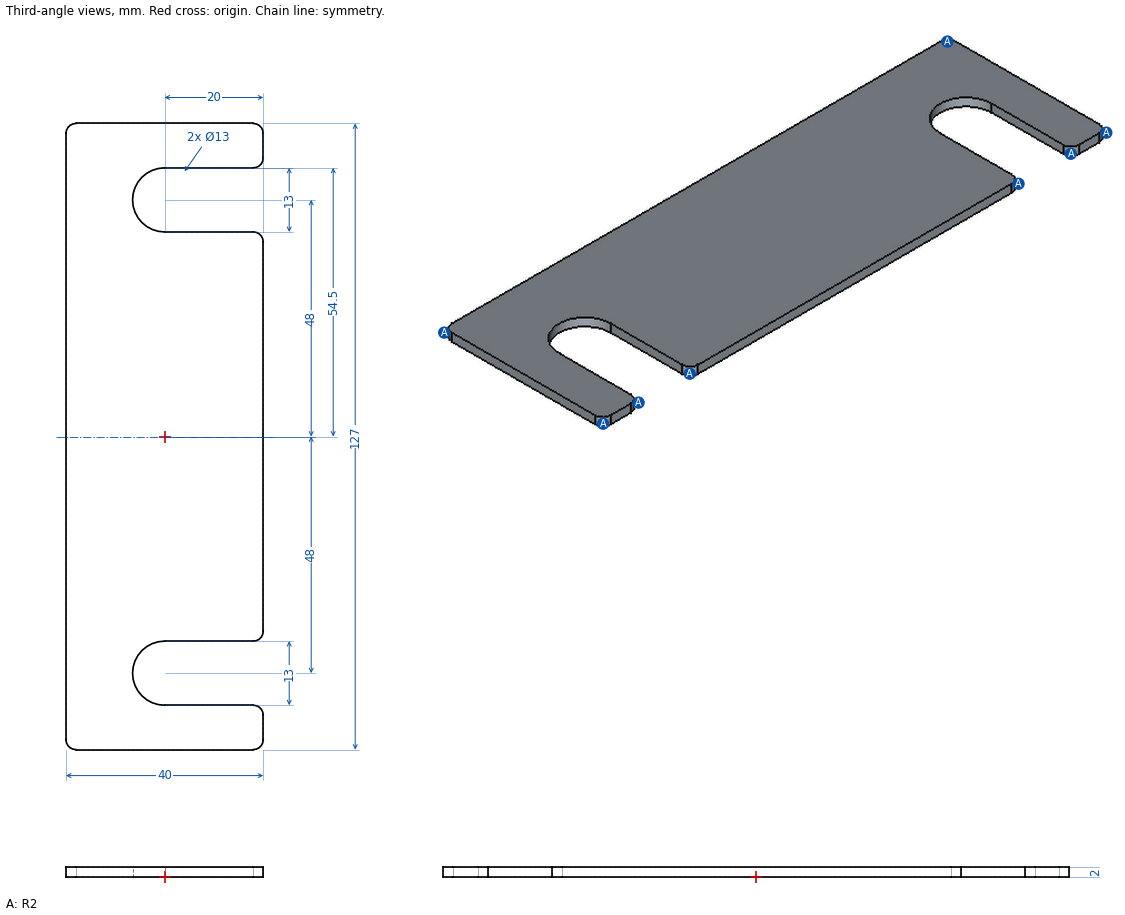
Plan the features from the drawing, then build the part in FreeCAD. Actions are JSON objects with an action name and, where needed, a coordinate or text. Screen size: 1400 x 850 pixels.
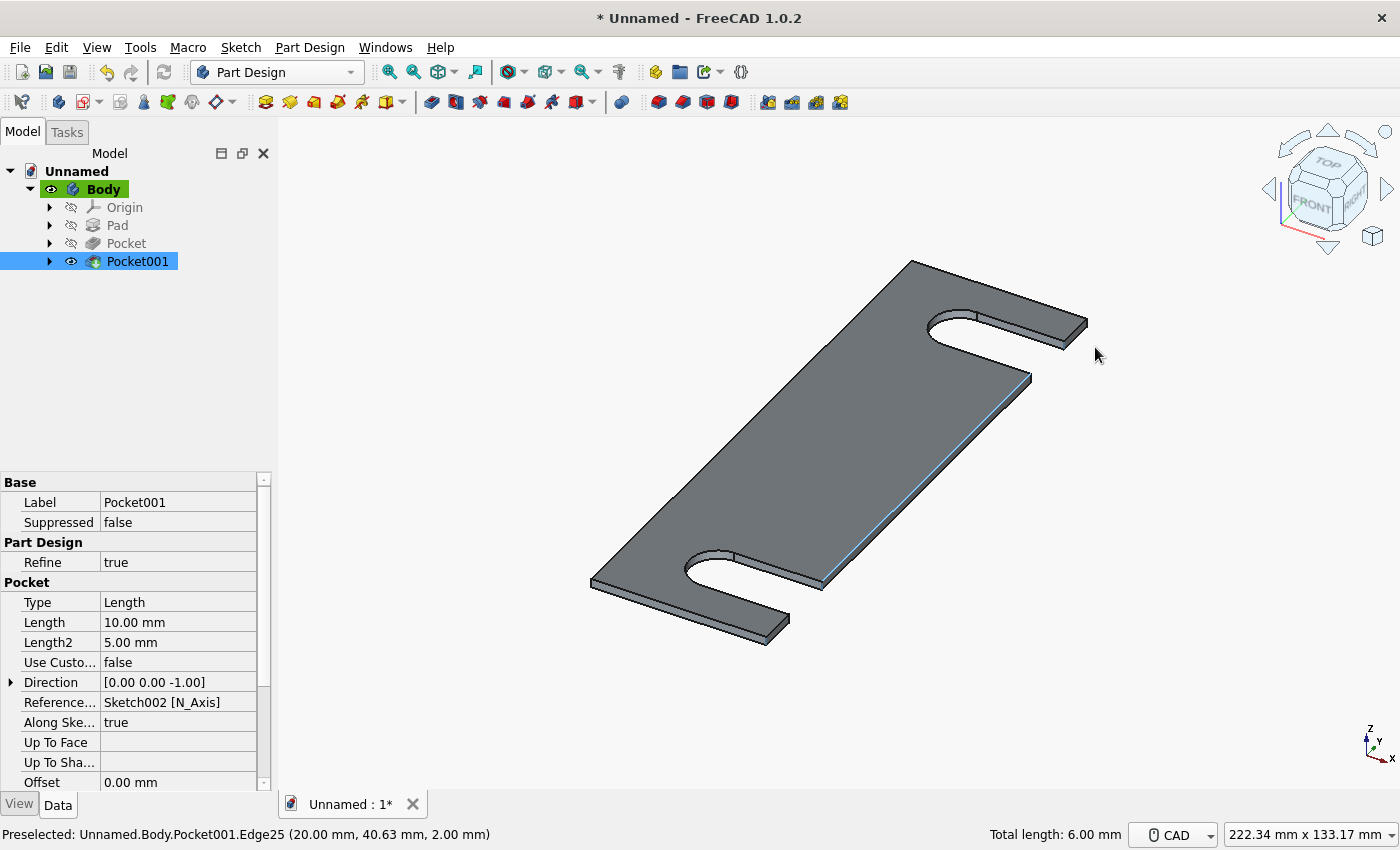
{"action": "key", "text": "0"}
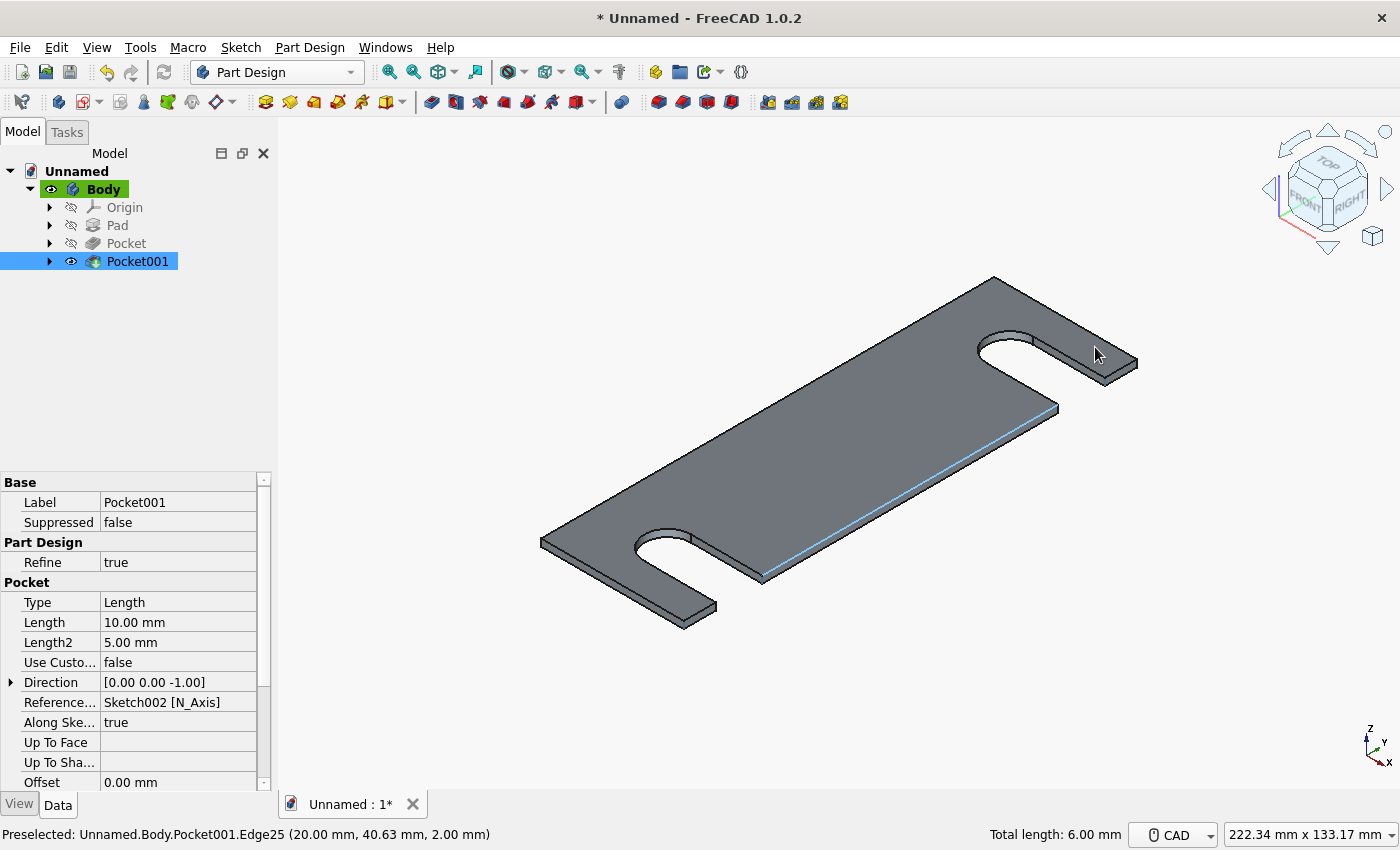
{"action": "scroll", "coordinate": [1058, 408], "scroll_direction": "up", "scroll_amount": 7}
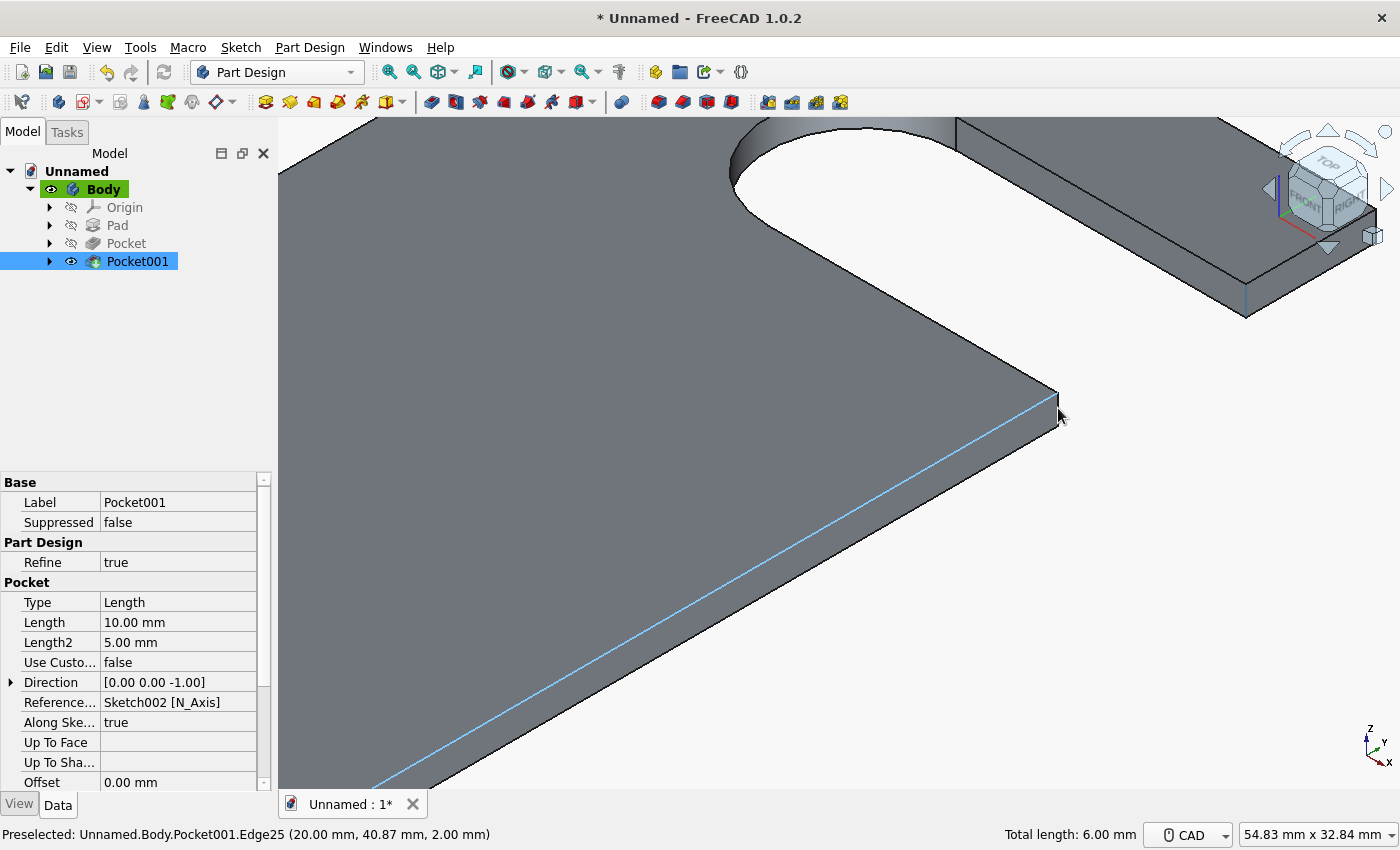
{"action": "left_click", "coordinate": [390, 72]}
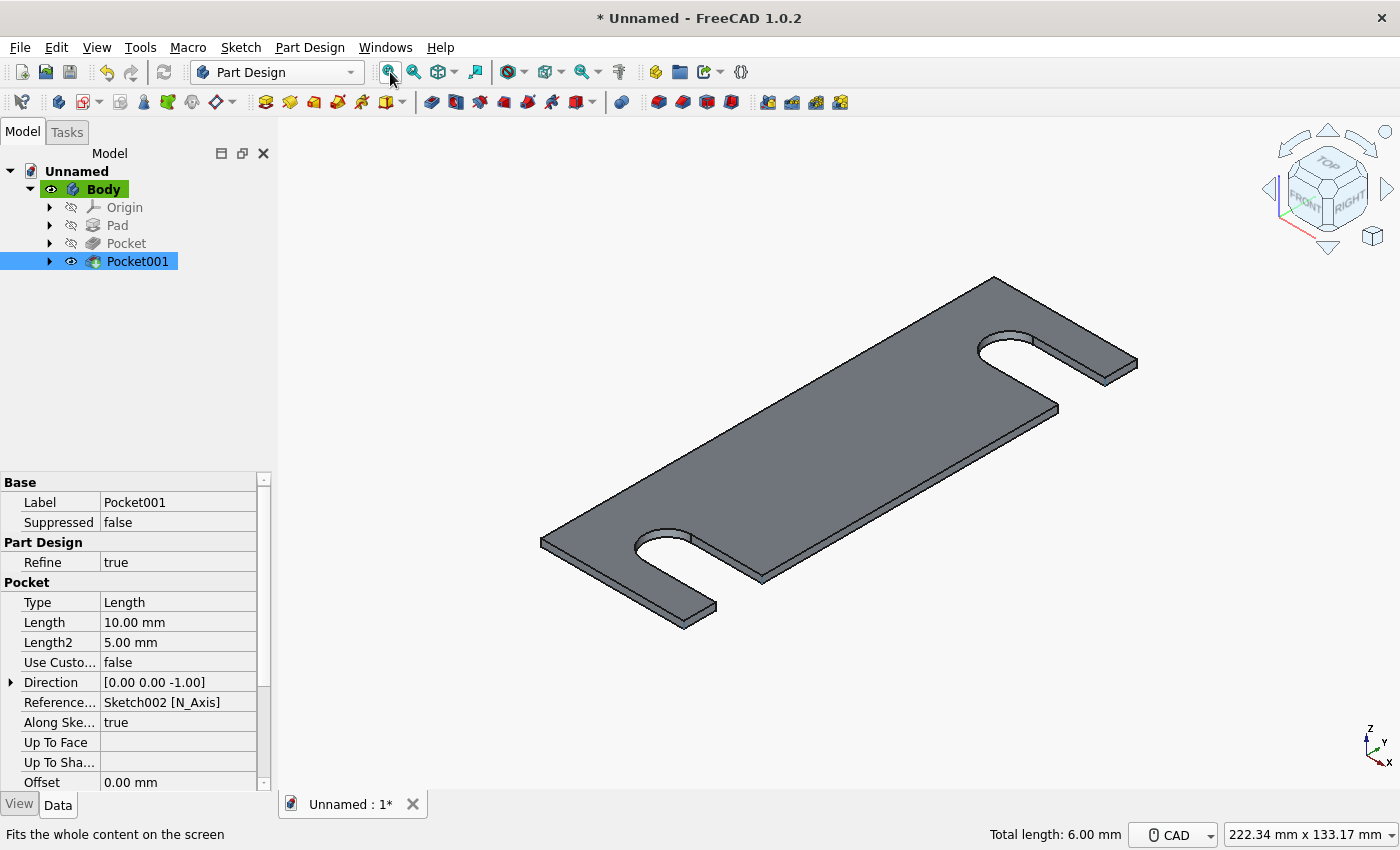
{"action": "key", "text": "2"}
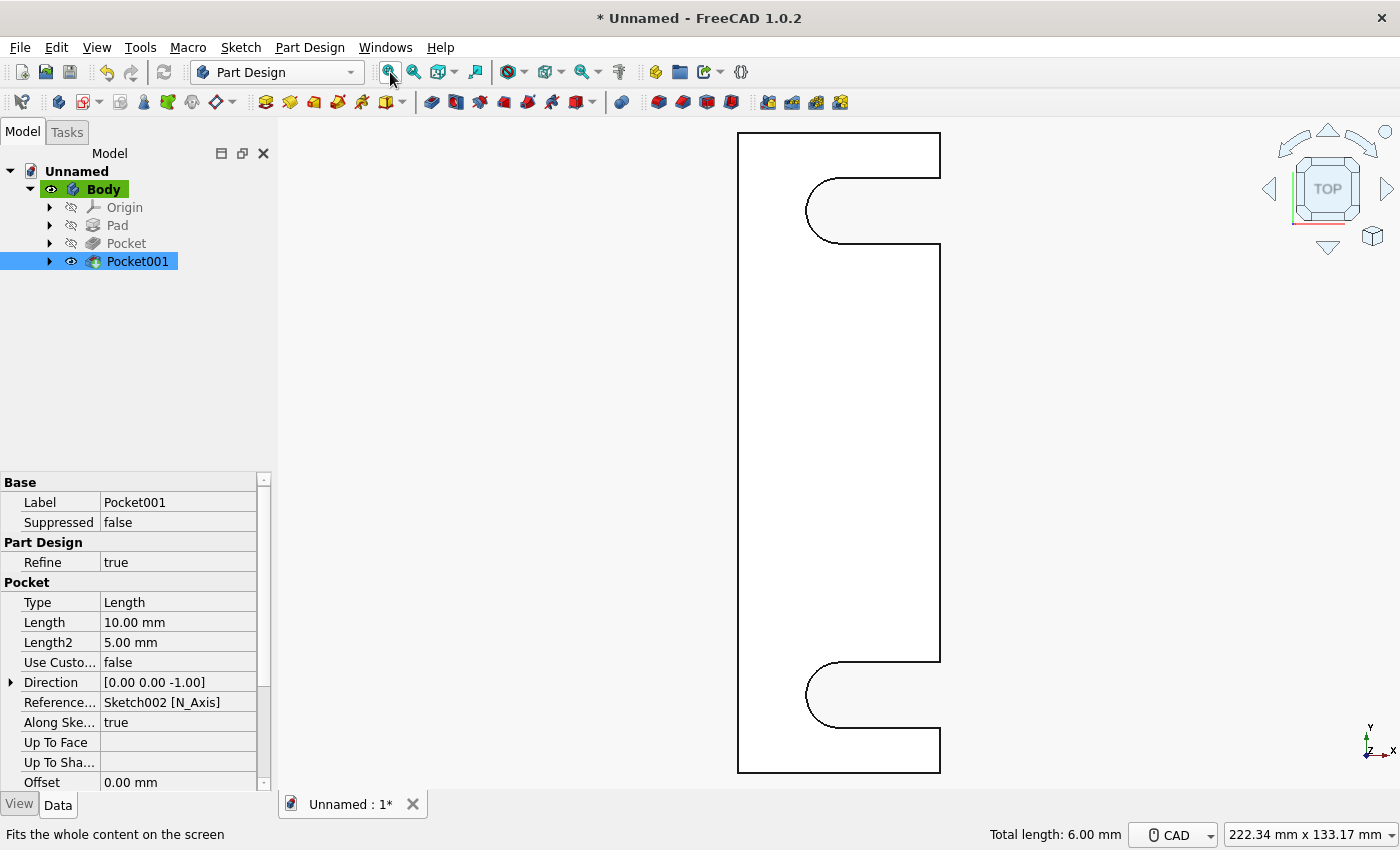
{"action": "scroll", "coordinate": [940, 243], "scroll_direction": "up", "scroll_amount": 7}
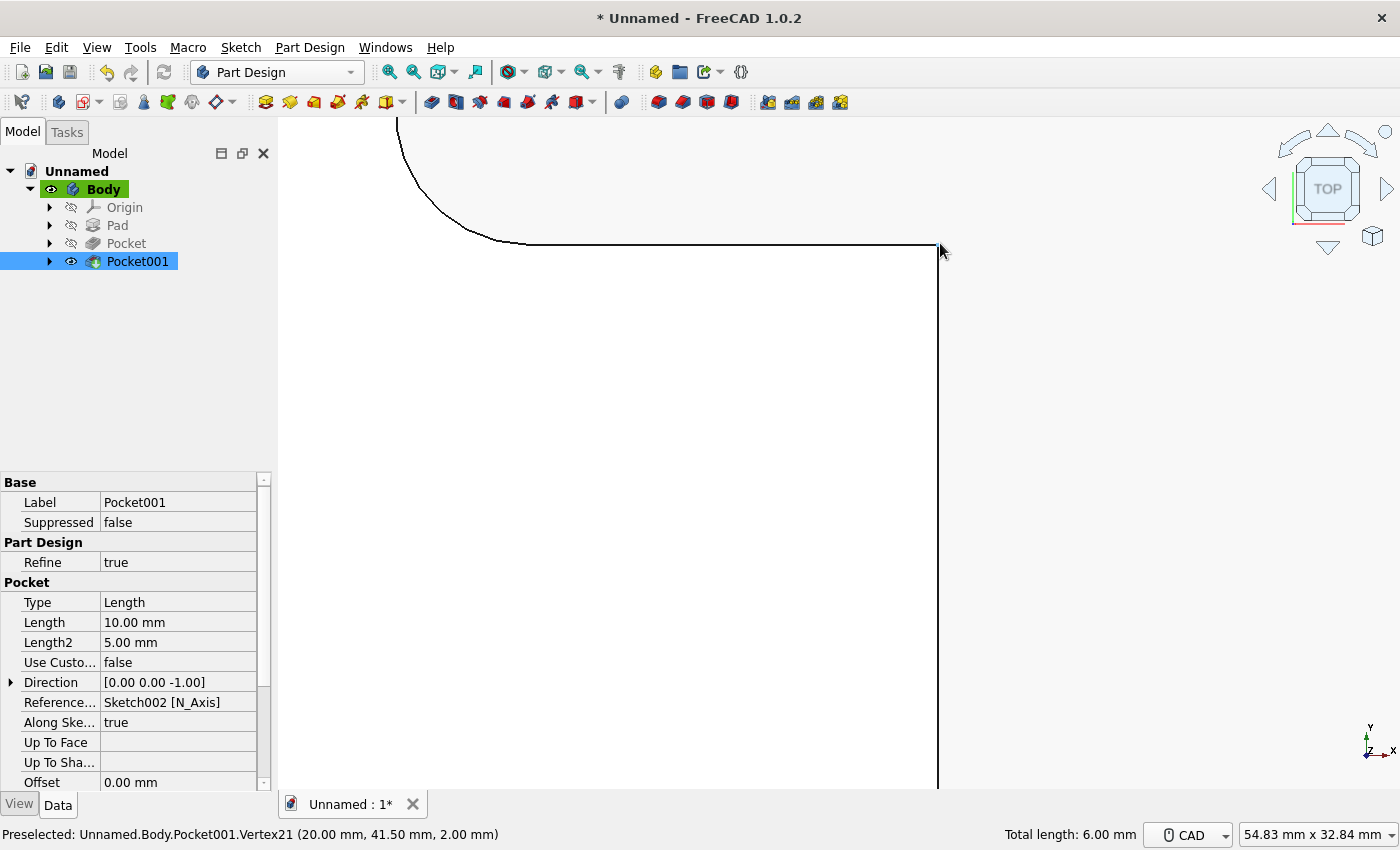
{"action": "left_click", "coordinate": [390, 72]}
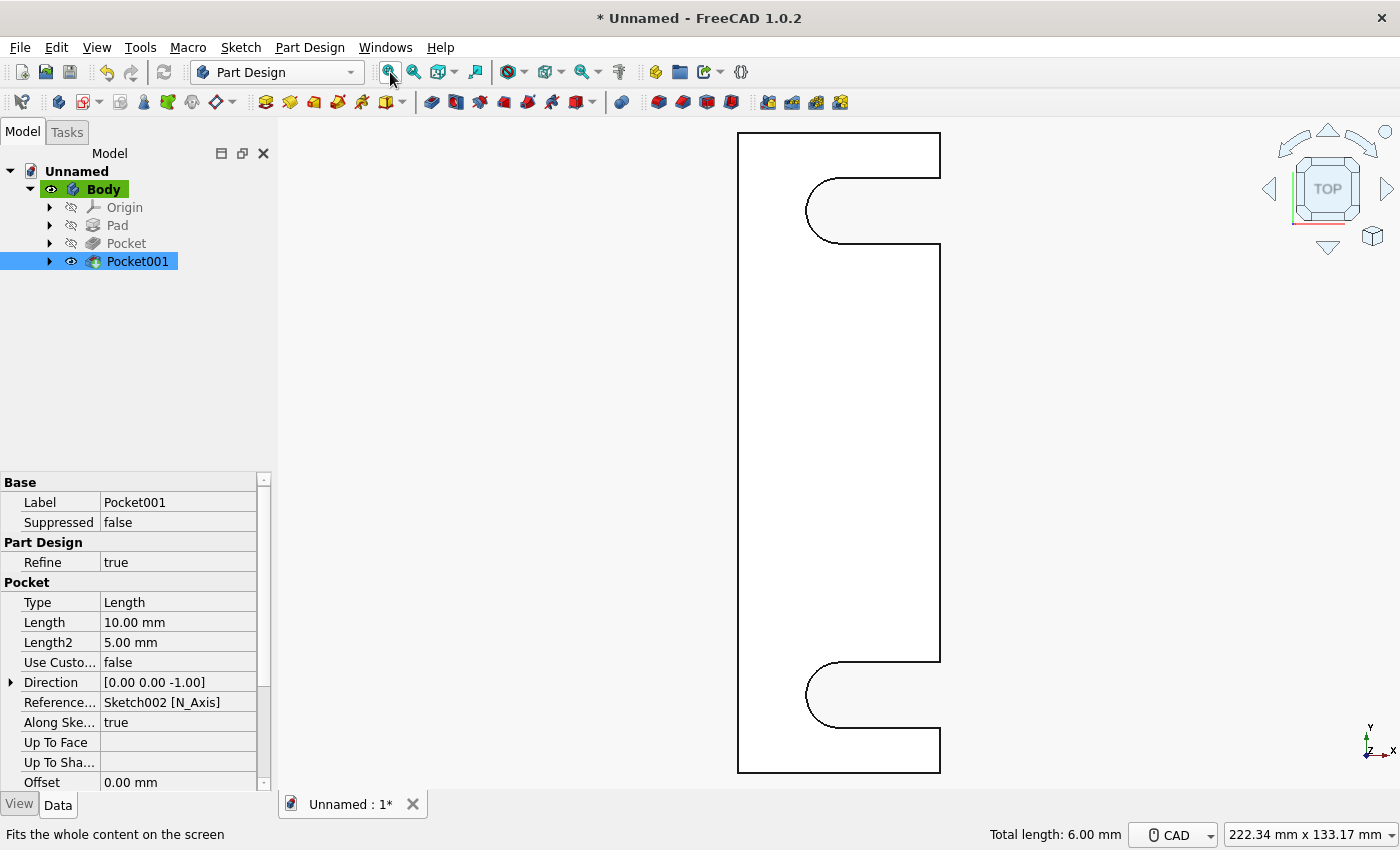
{"action": "key", "text": "1"}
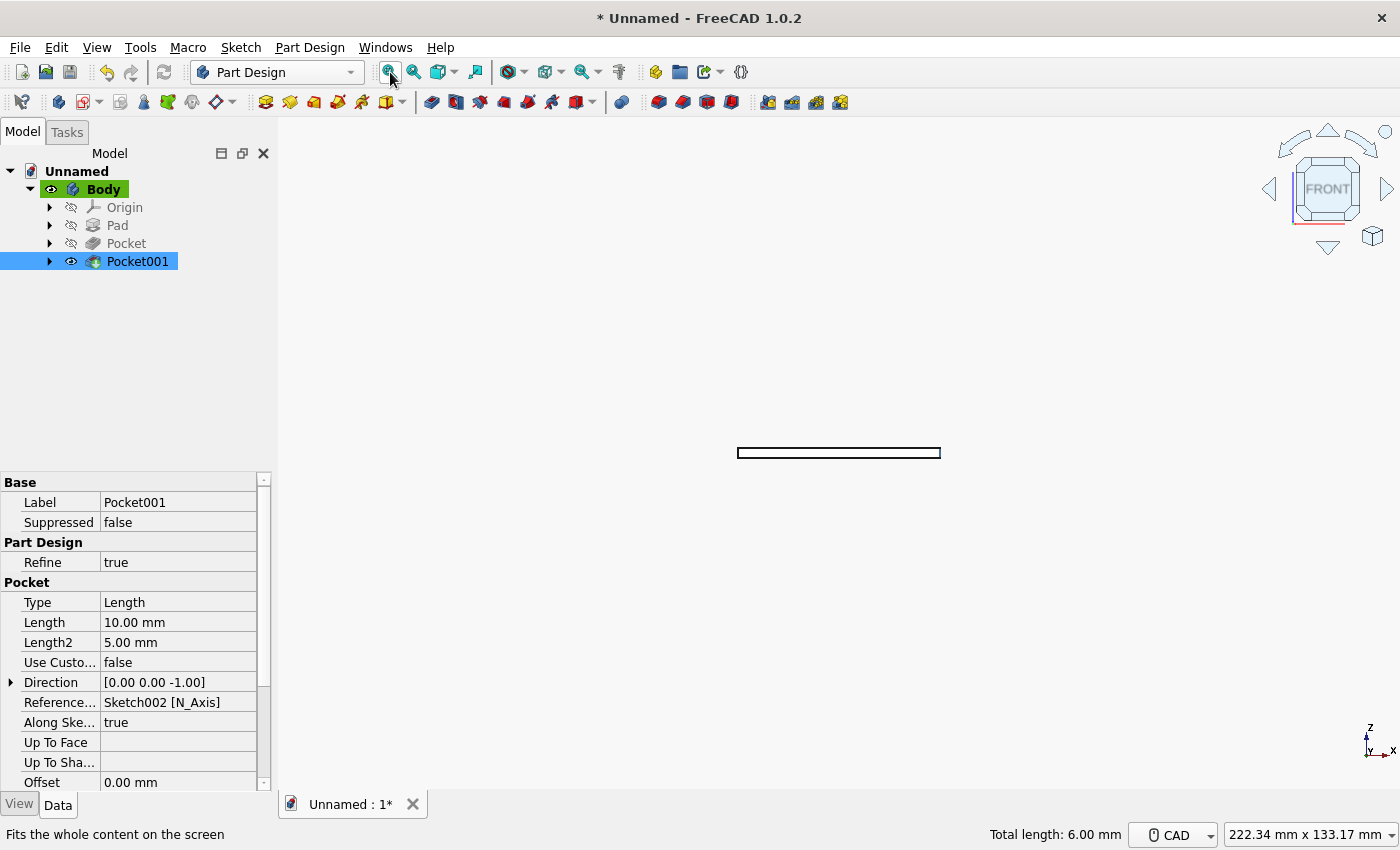
{"action": "left_click", "coordinate": [390, 72]}